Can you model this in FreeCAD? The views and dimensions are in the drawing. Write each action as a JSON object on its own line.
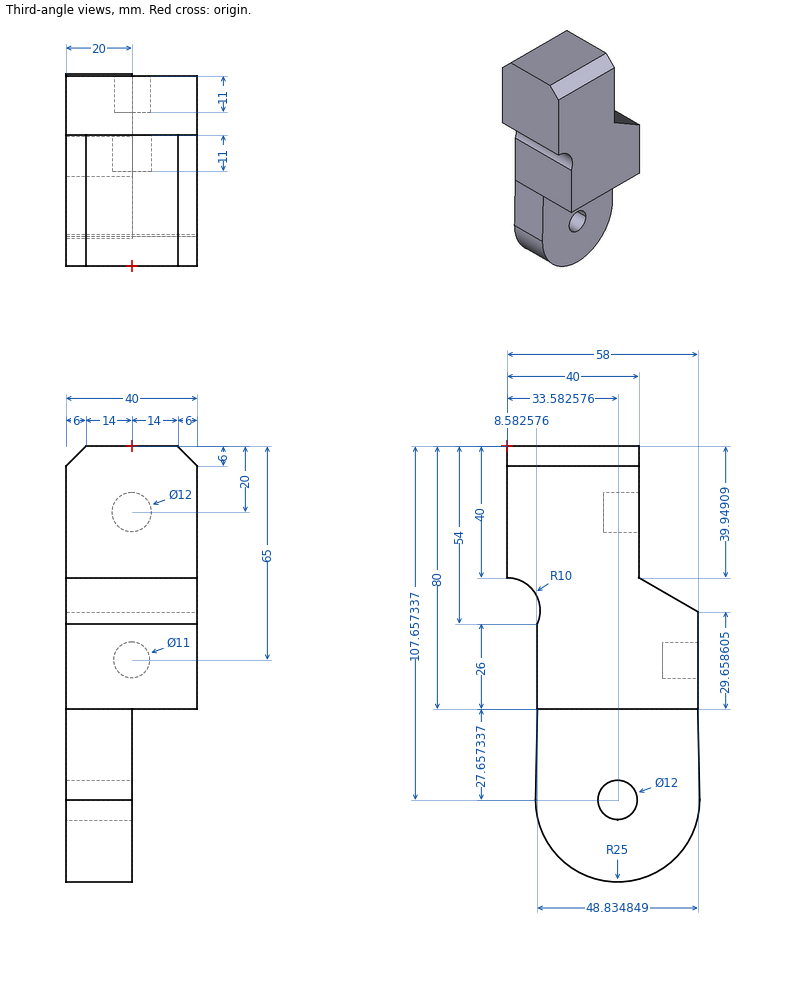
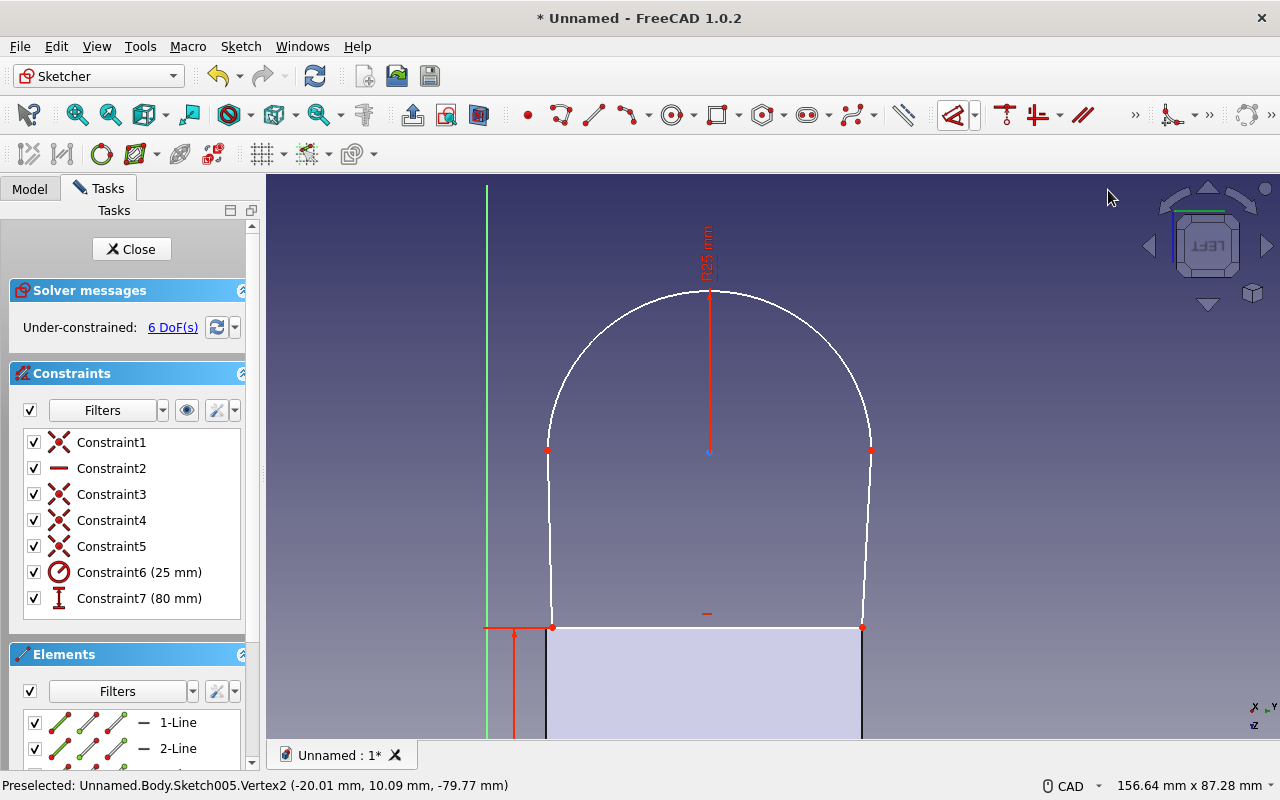
{"action": "left_click", "coordinate": [862, 628]}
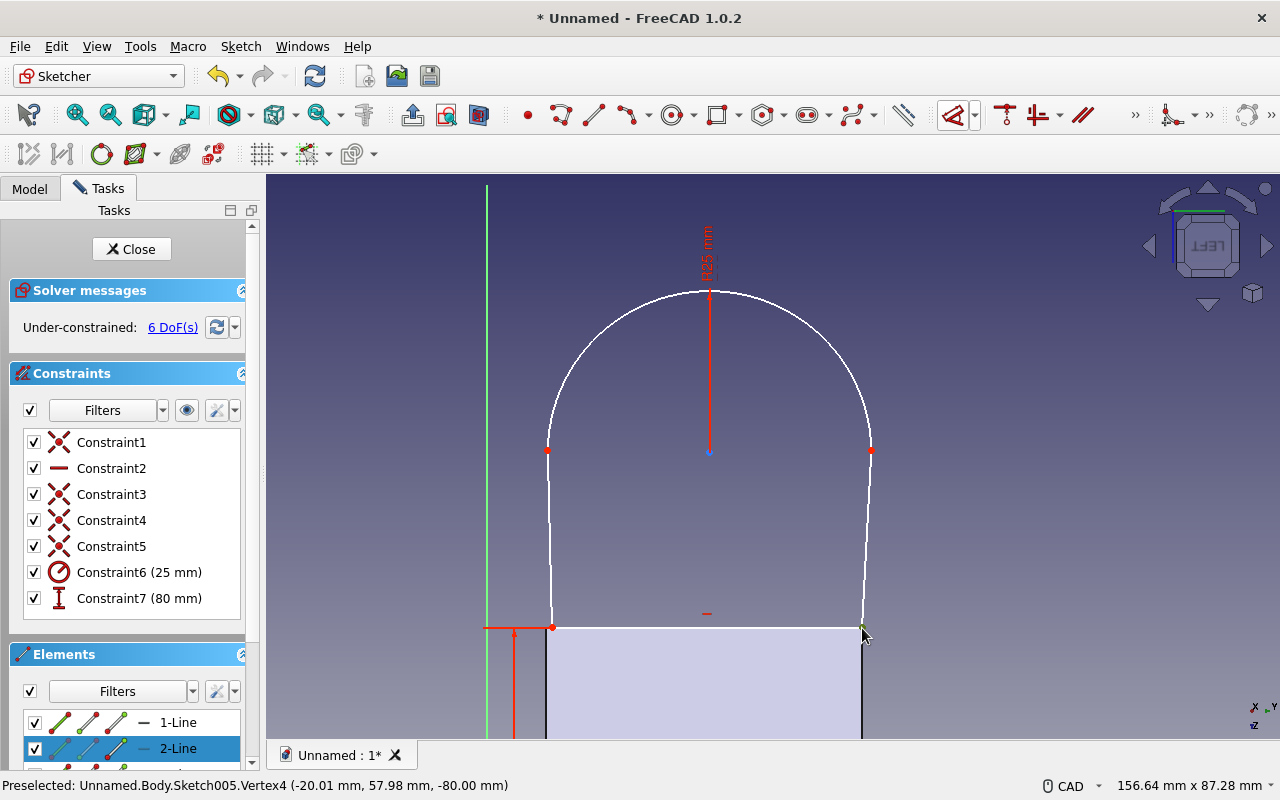
{"action": "key", "text": "l"}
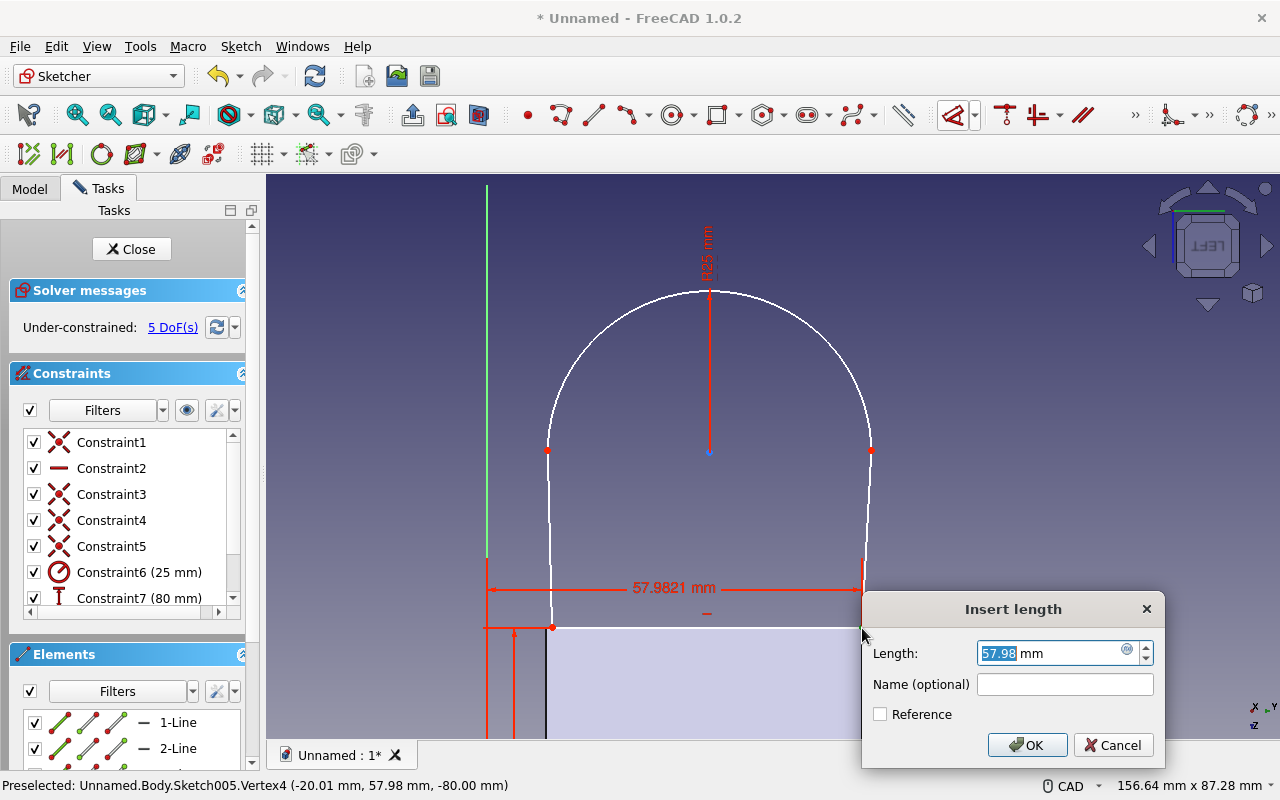
{"action": "type", "text": "58"}
{"action": "key", "text": "Return"}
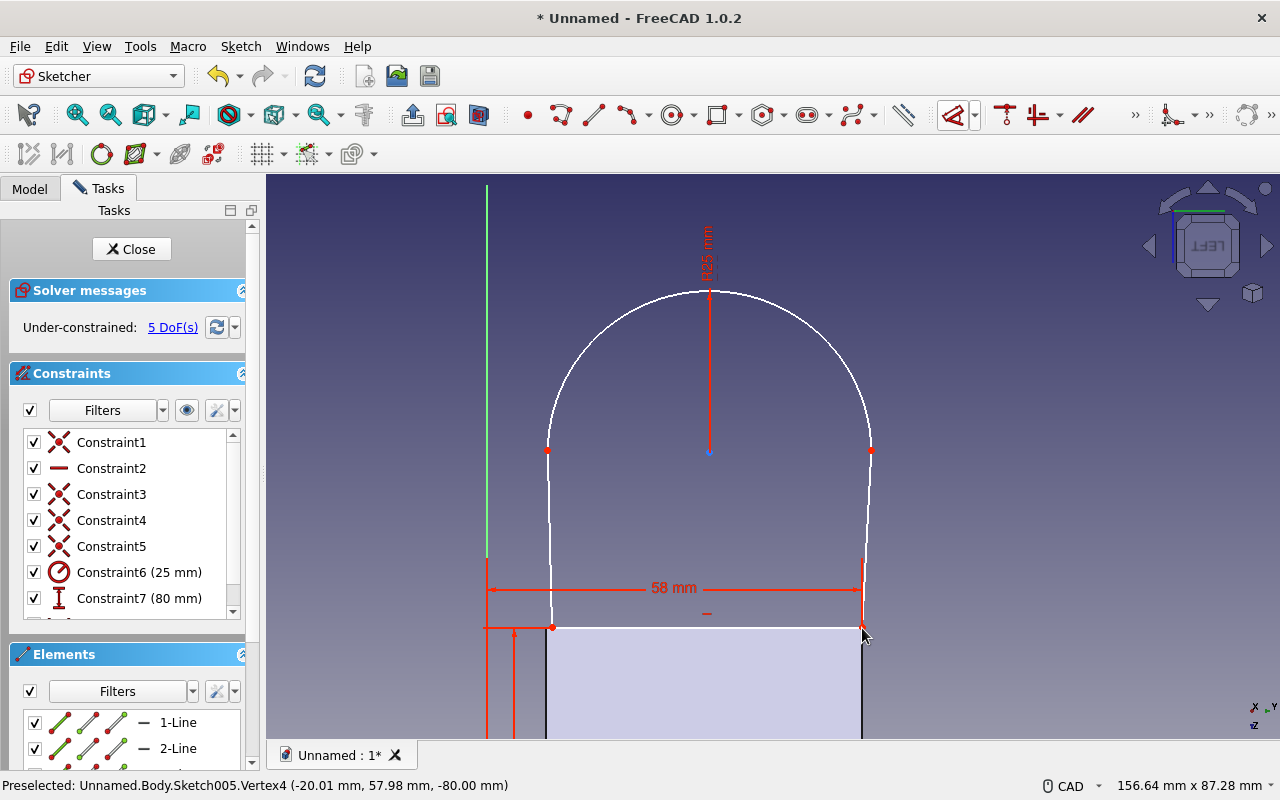
{"action": "left_click", "coordinate": [645, 628]}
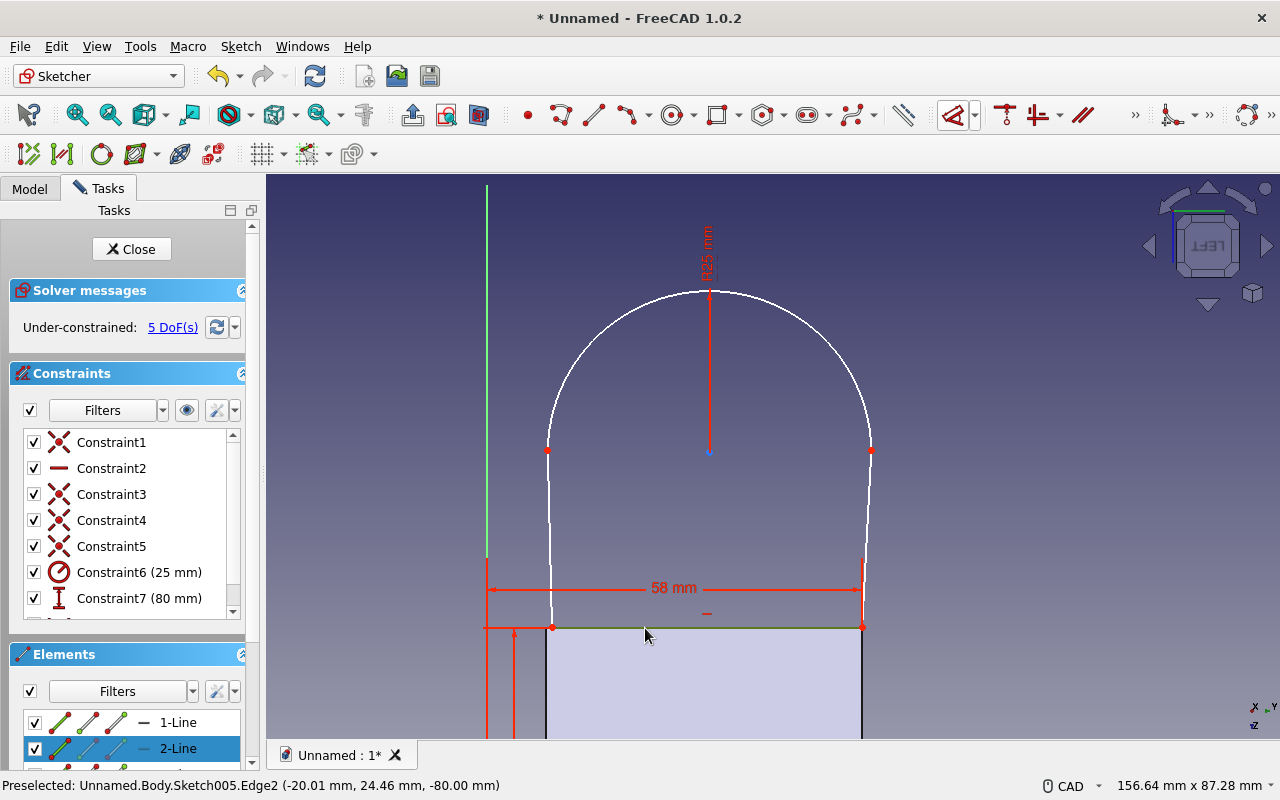
{"action": "left_click", "coordinate": [974, 116]}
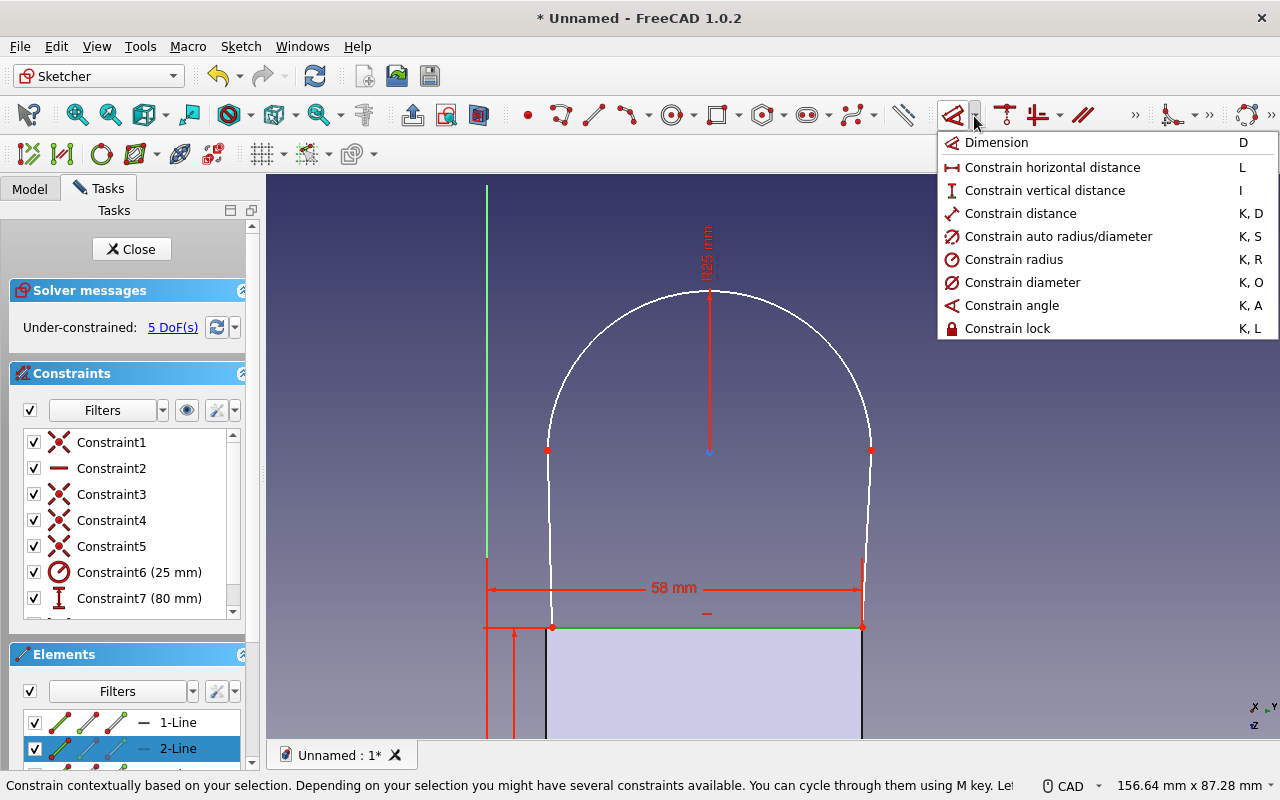
{"action": "left_click", "coordinate": [1108, 168]}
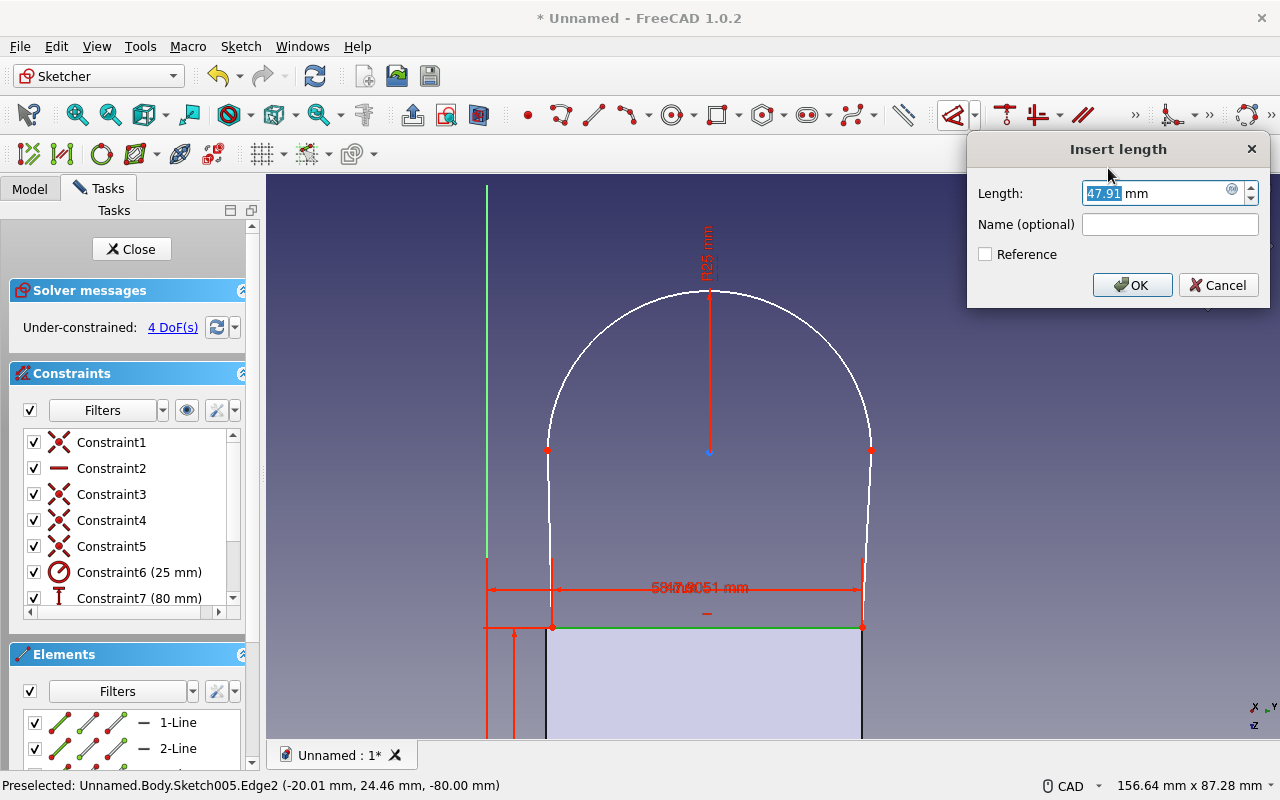
{"action": "type", "text": "48.834849"}
{"action": "key", "text": "Return"}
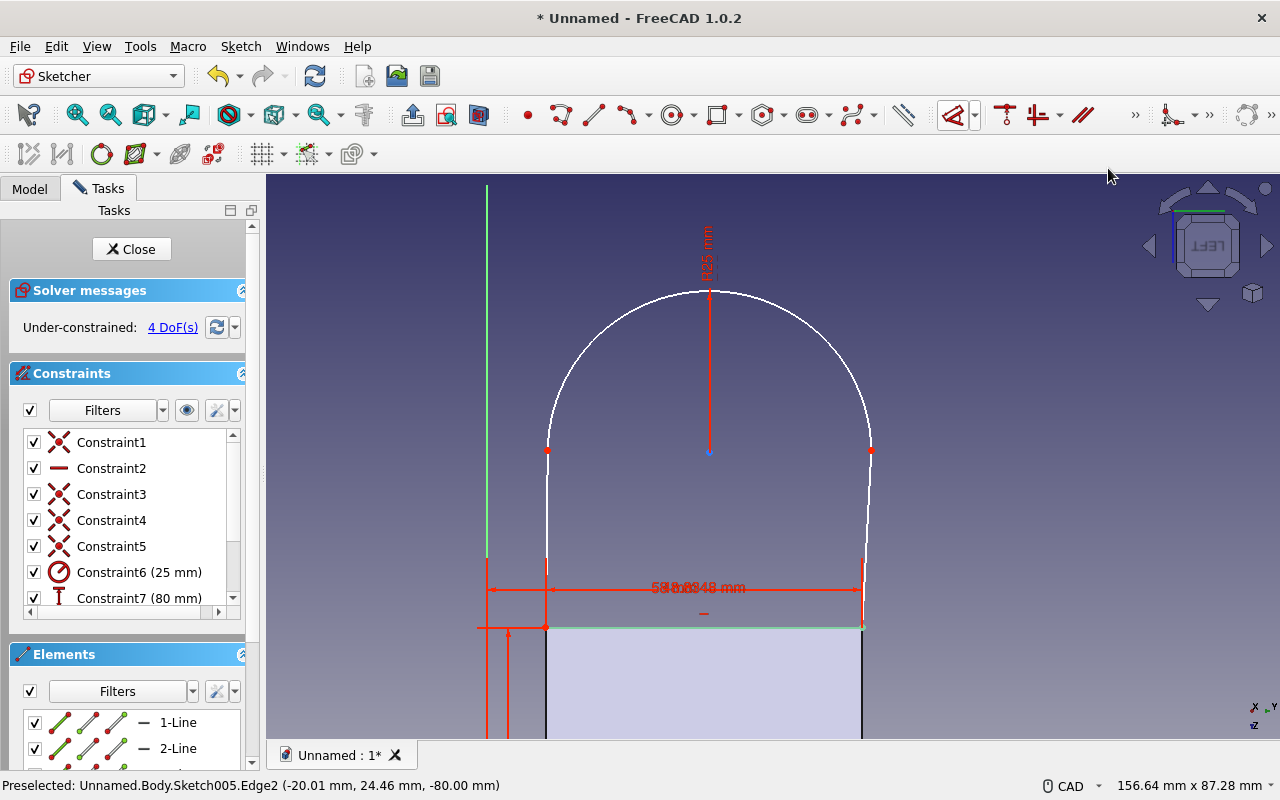
{"action": "left_click", "coordinate": [548, 450]}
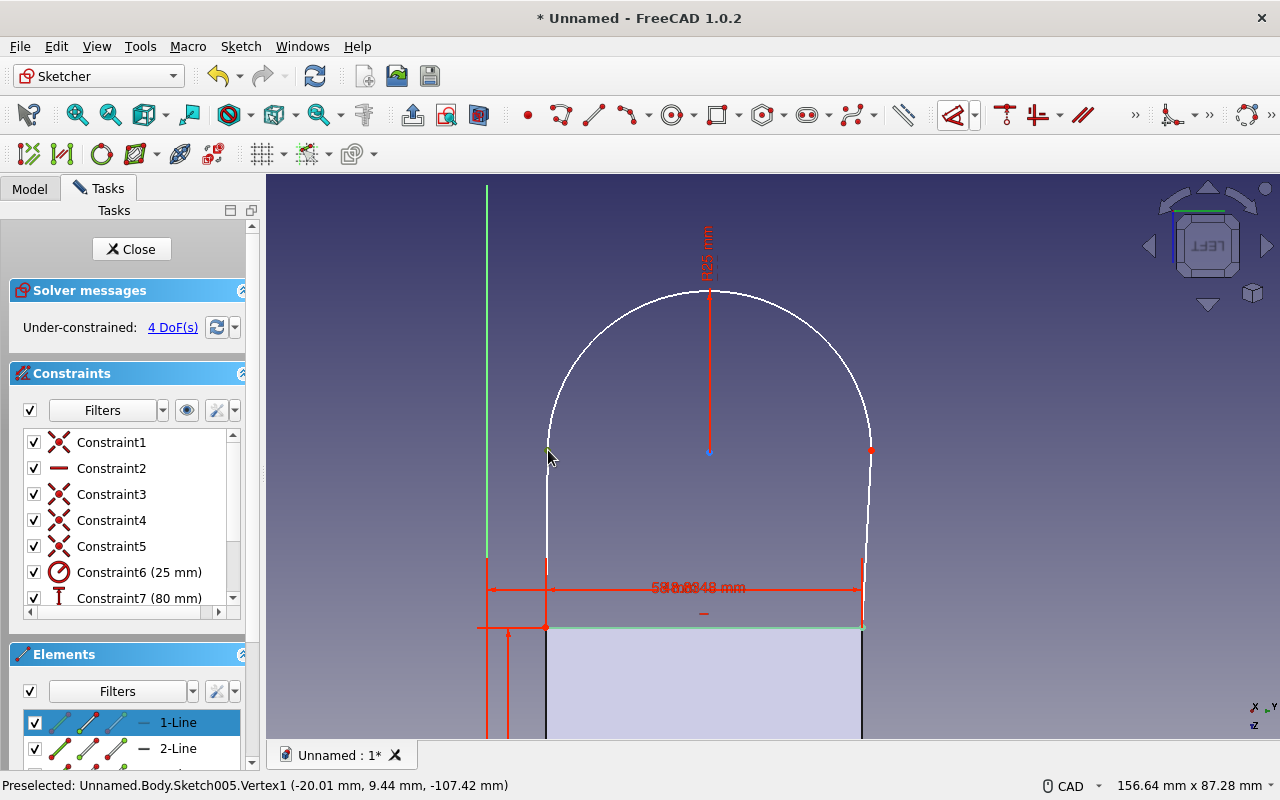
{"action": "left_click", "coordinate": [974, 116]}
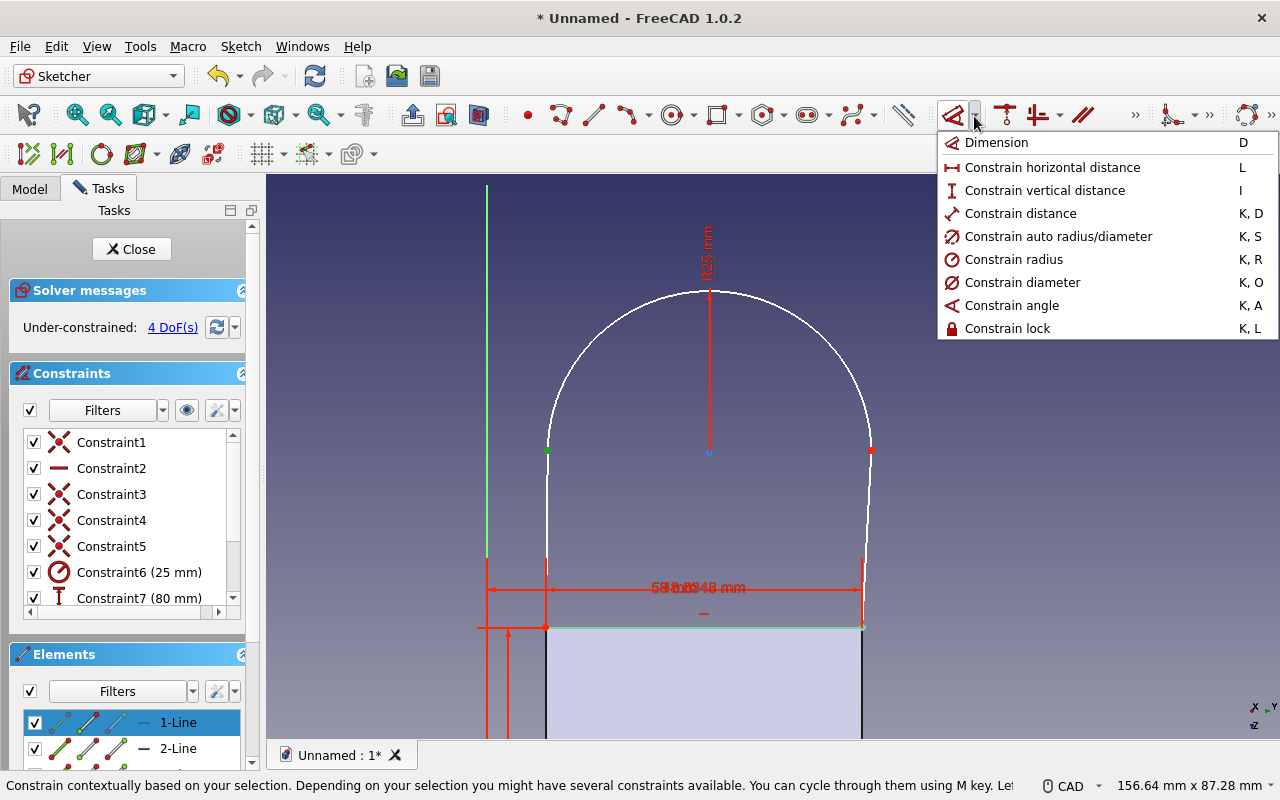
{"action": "left_click", "coordinate": [1108, 168]}